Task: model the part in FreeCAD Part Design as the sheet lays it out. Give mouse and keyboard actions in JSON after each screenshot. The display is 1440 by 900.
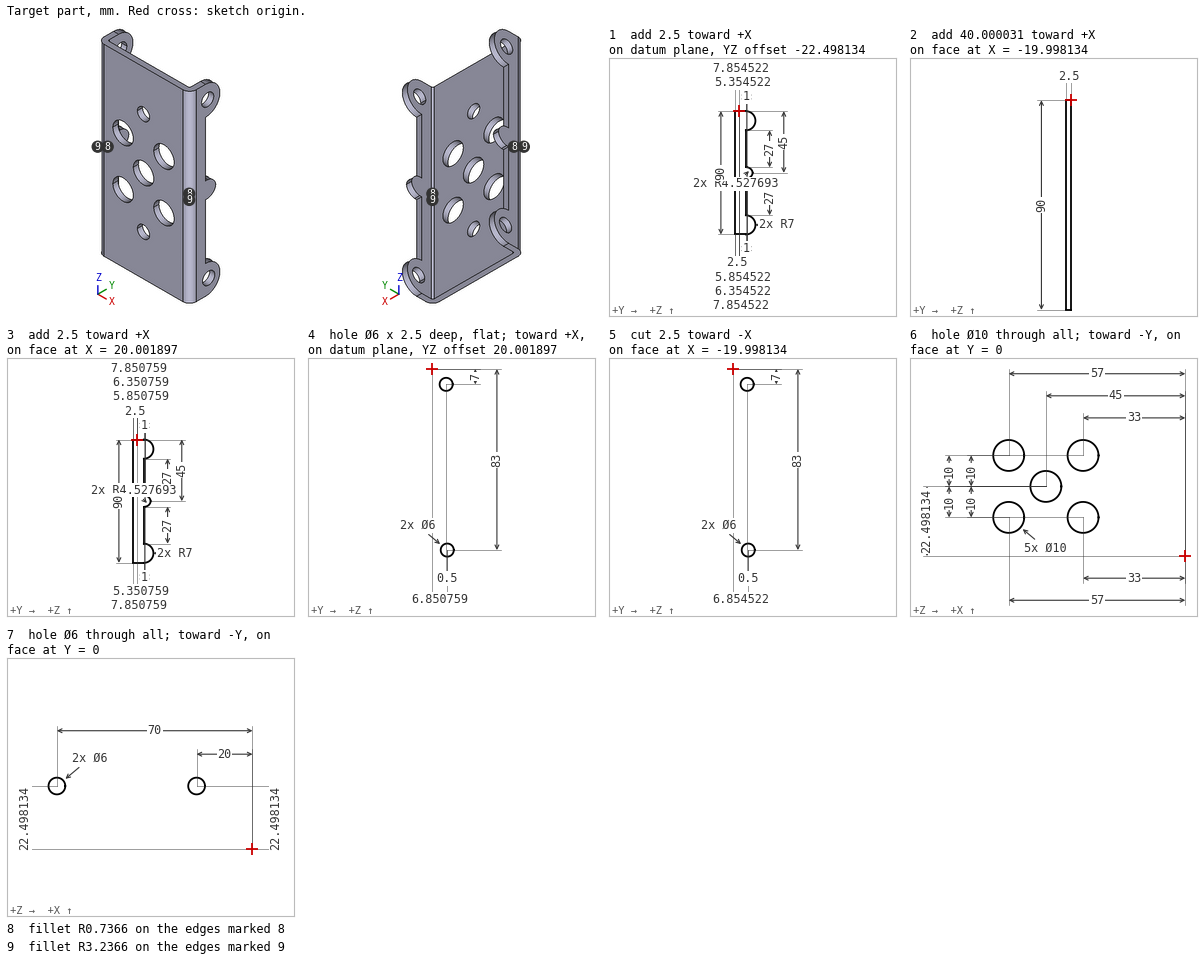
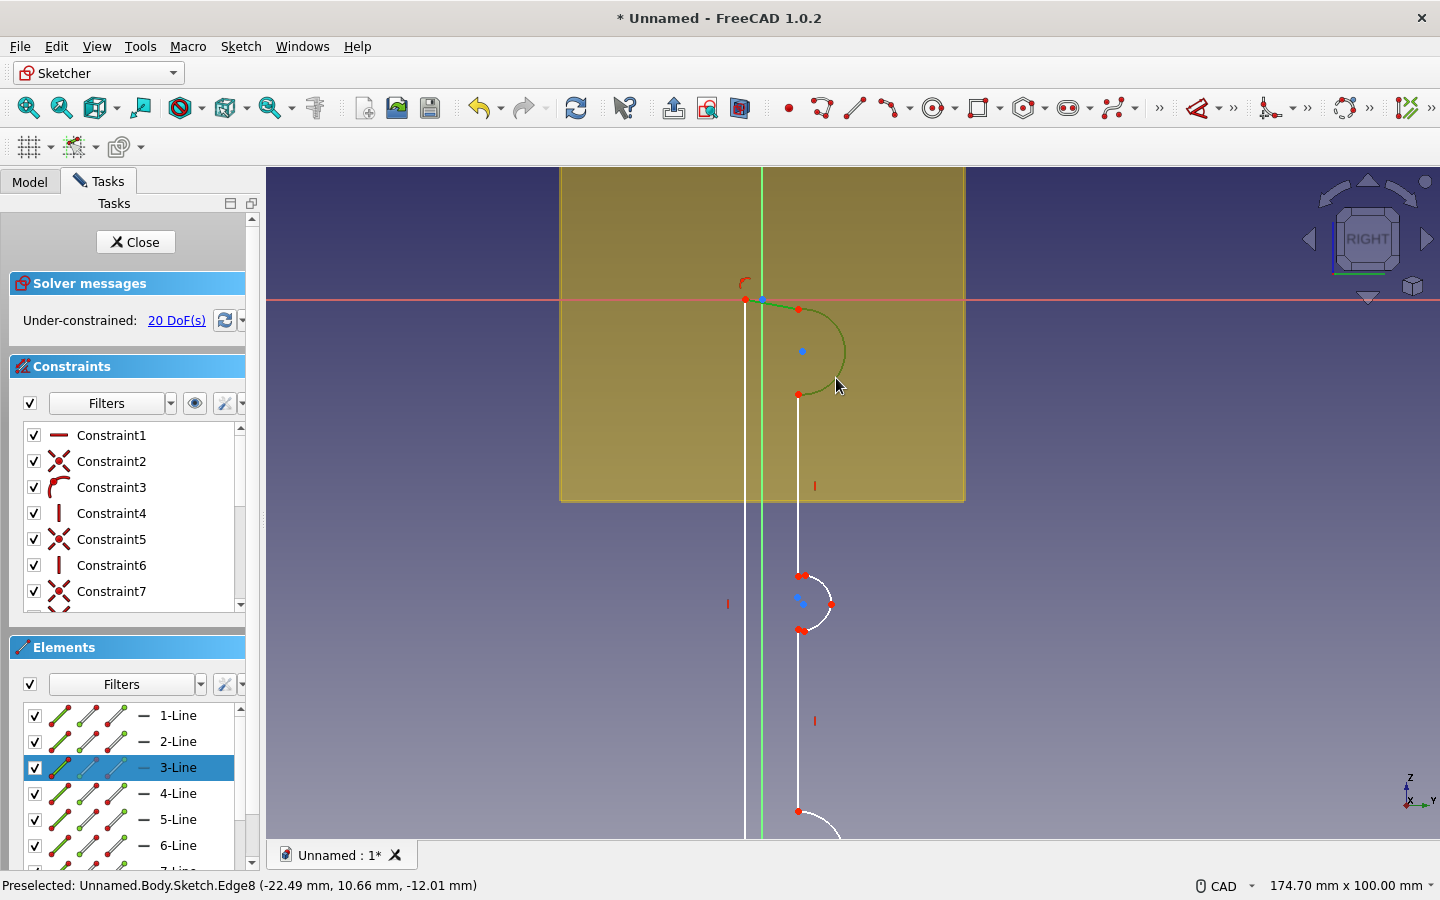
{"action": "key", "text": "t"}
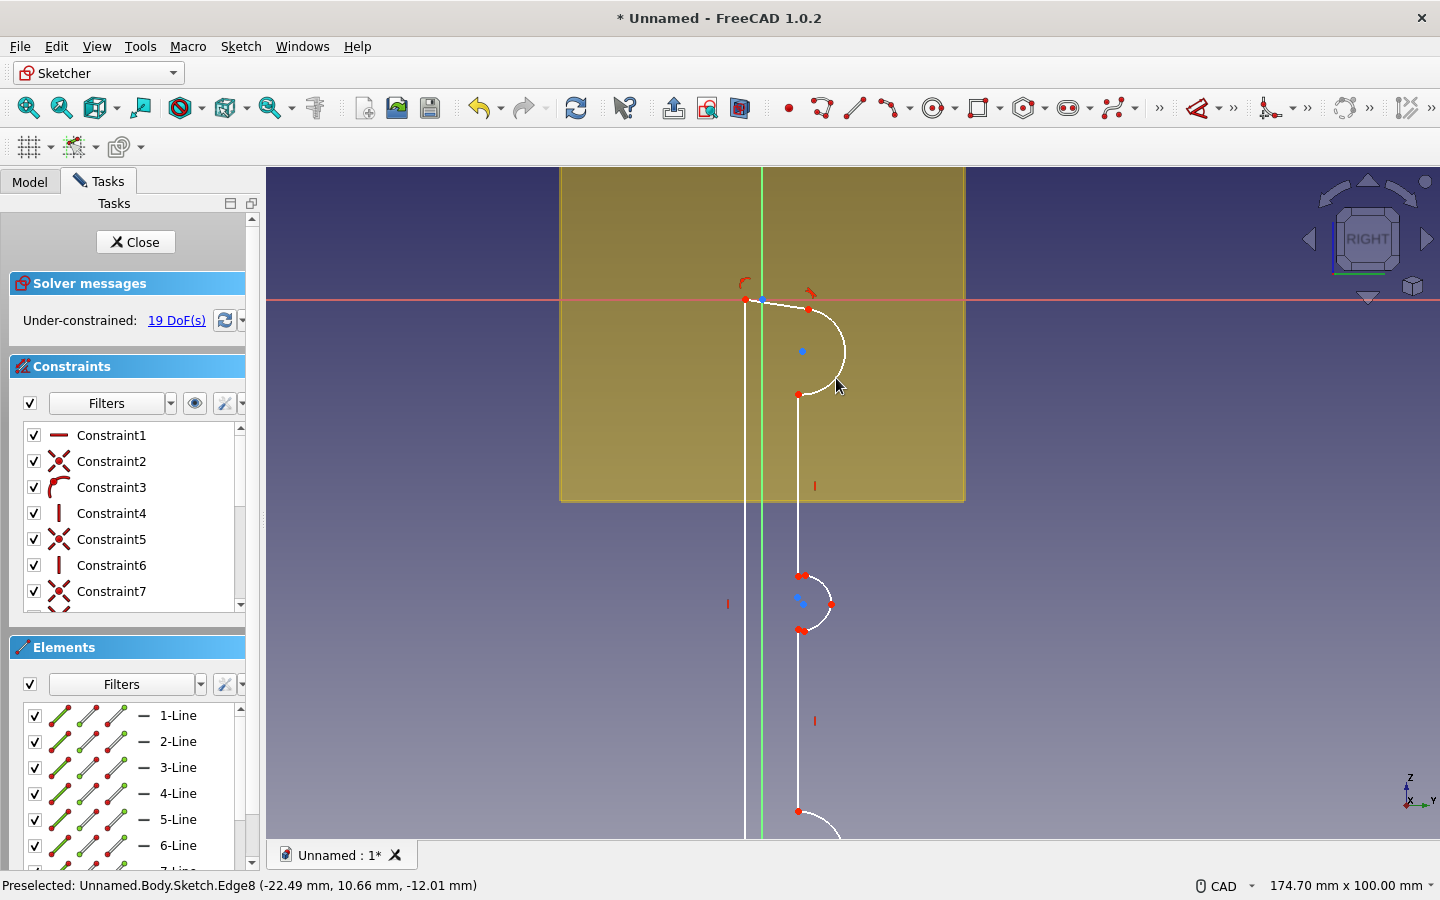
{"action": "left_click", "coordinate": [771, 304]}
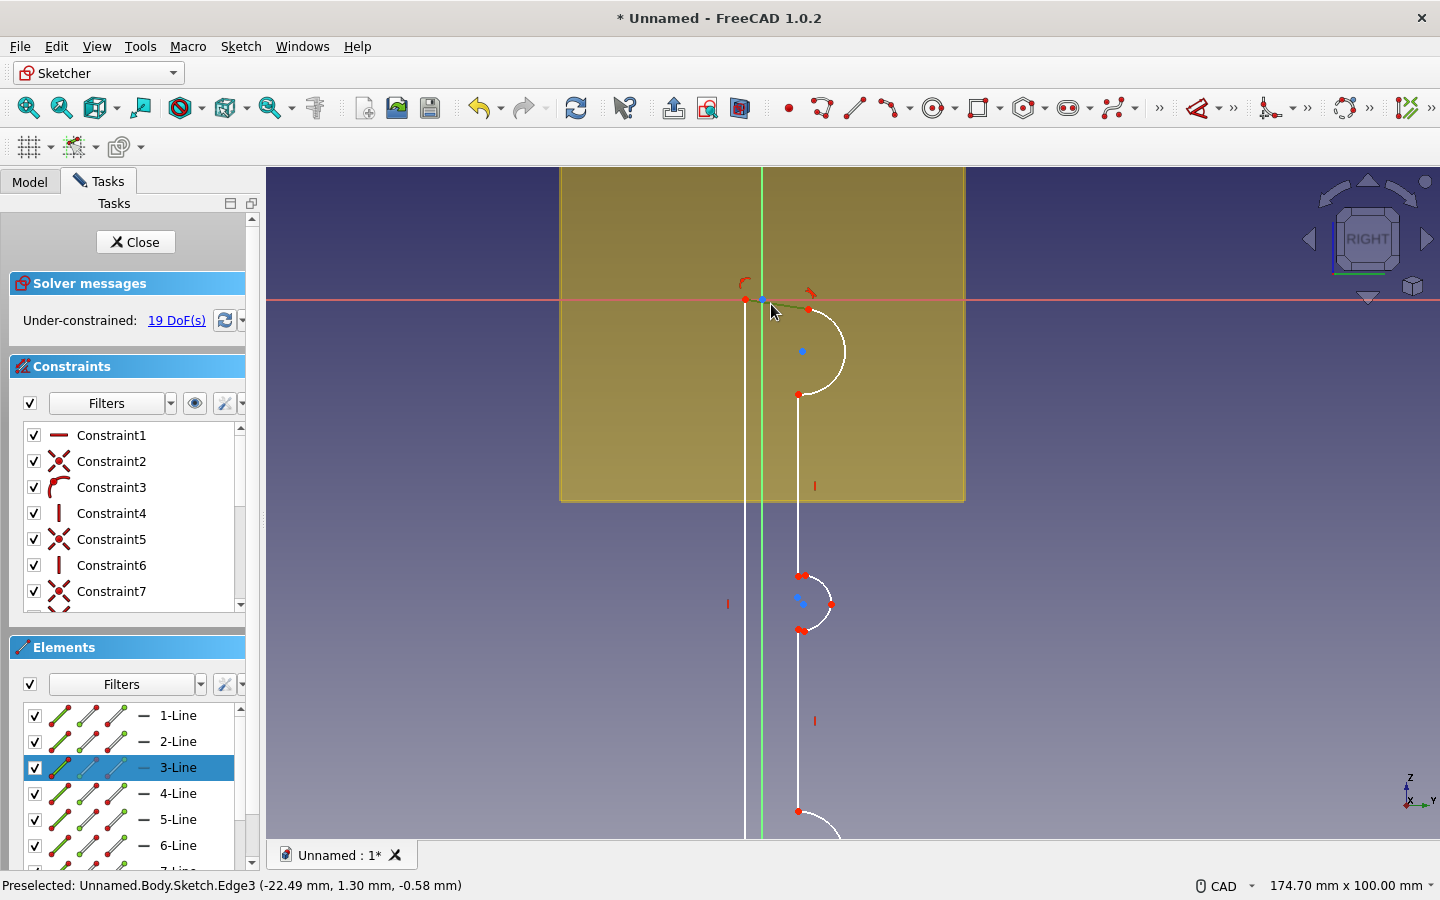
{"action": "key", "text": "h"}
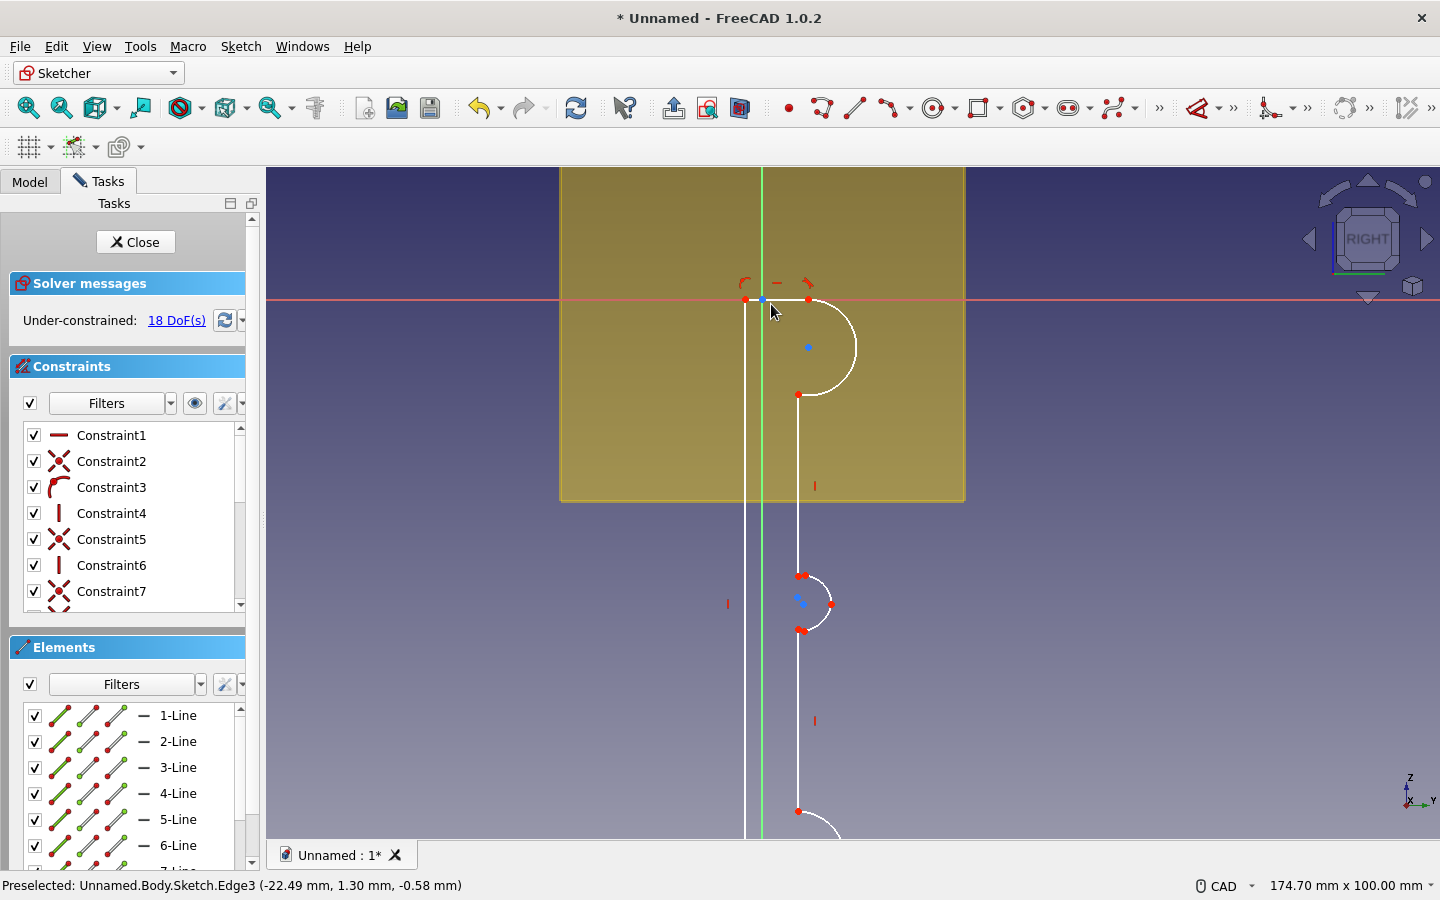
{"action": "scroll", "coordinate": [802, 576], "scroll_direction": "up", "scroll_amount": 7}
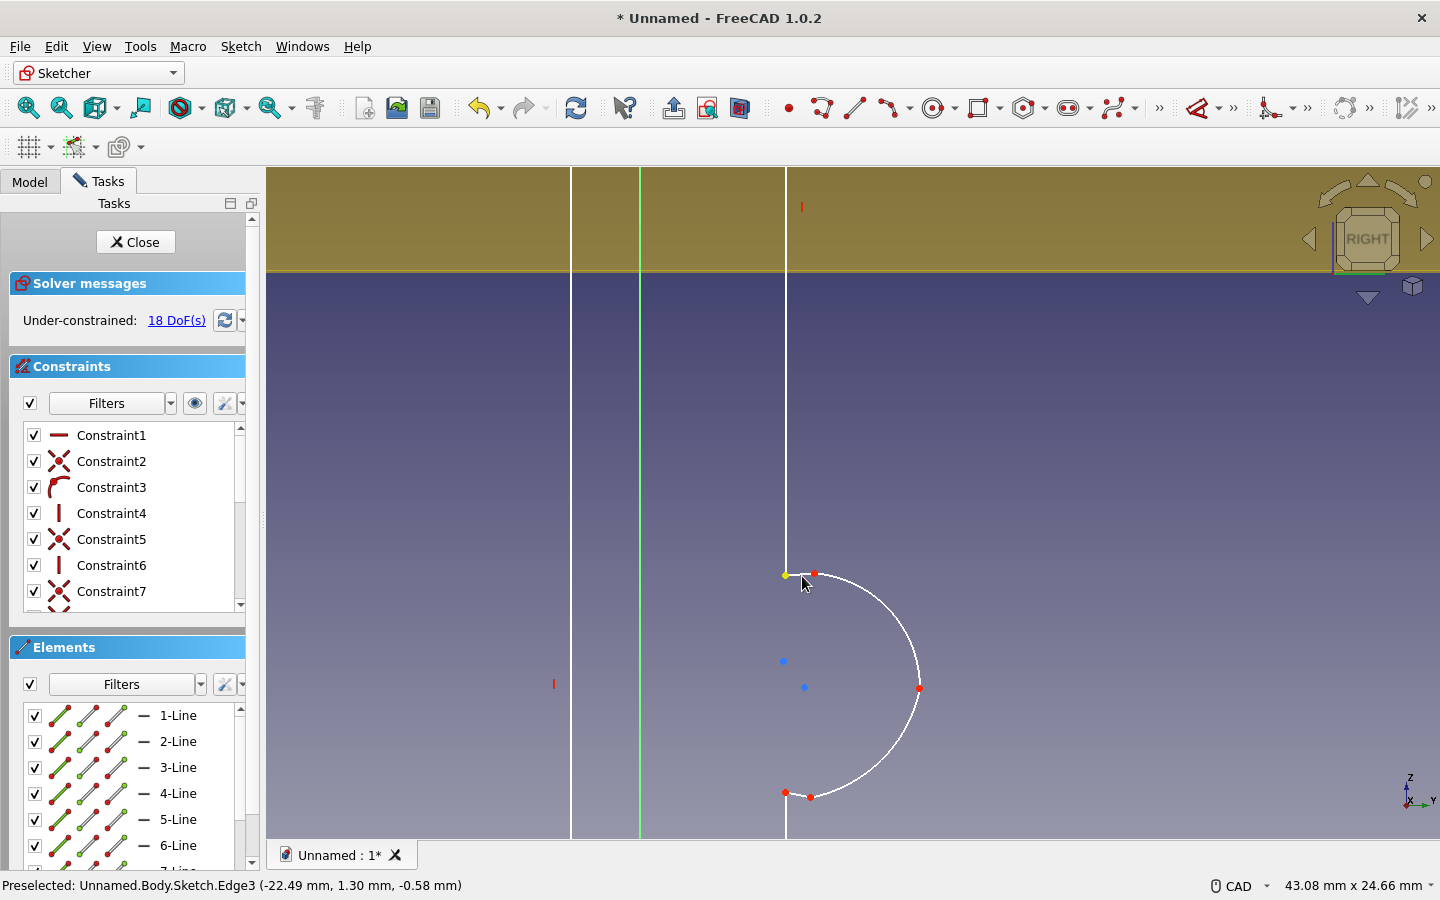
{"action": "left_click", "coordinate": [800, 574]}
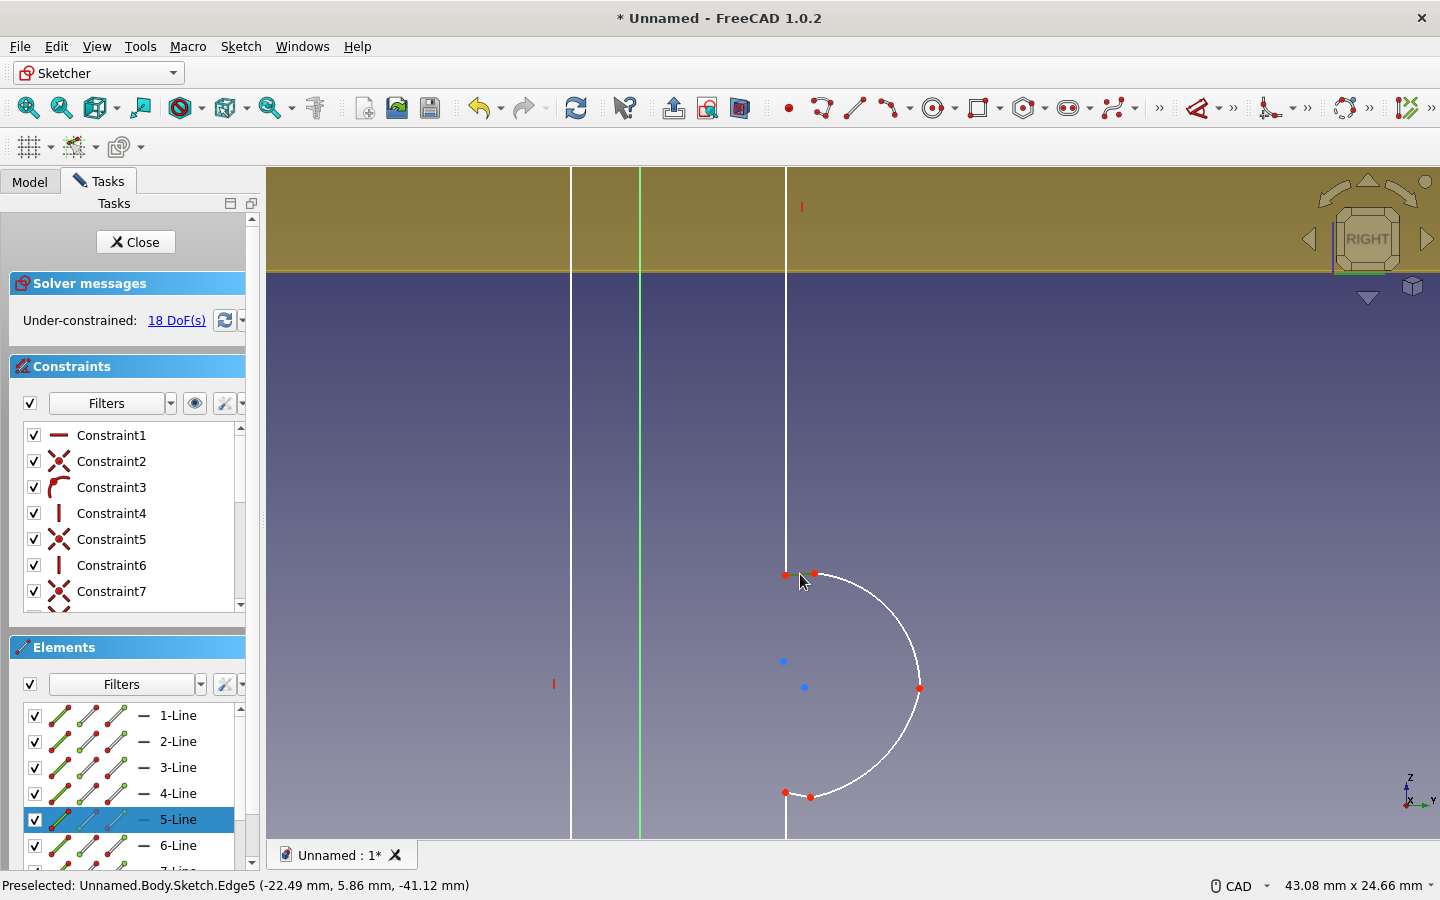
{"action": "key", "text": "h"}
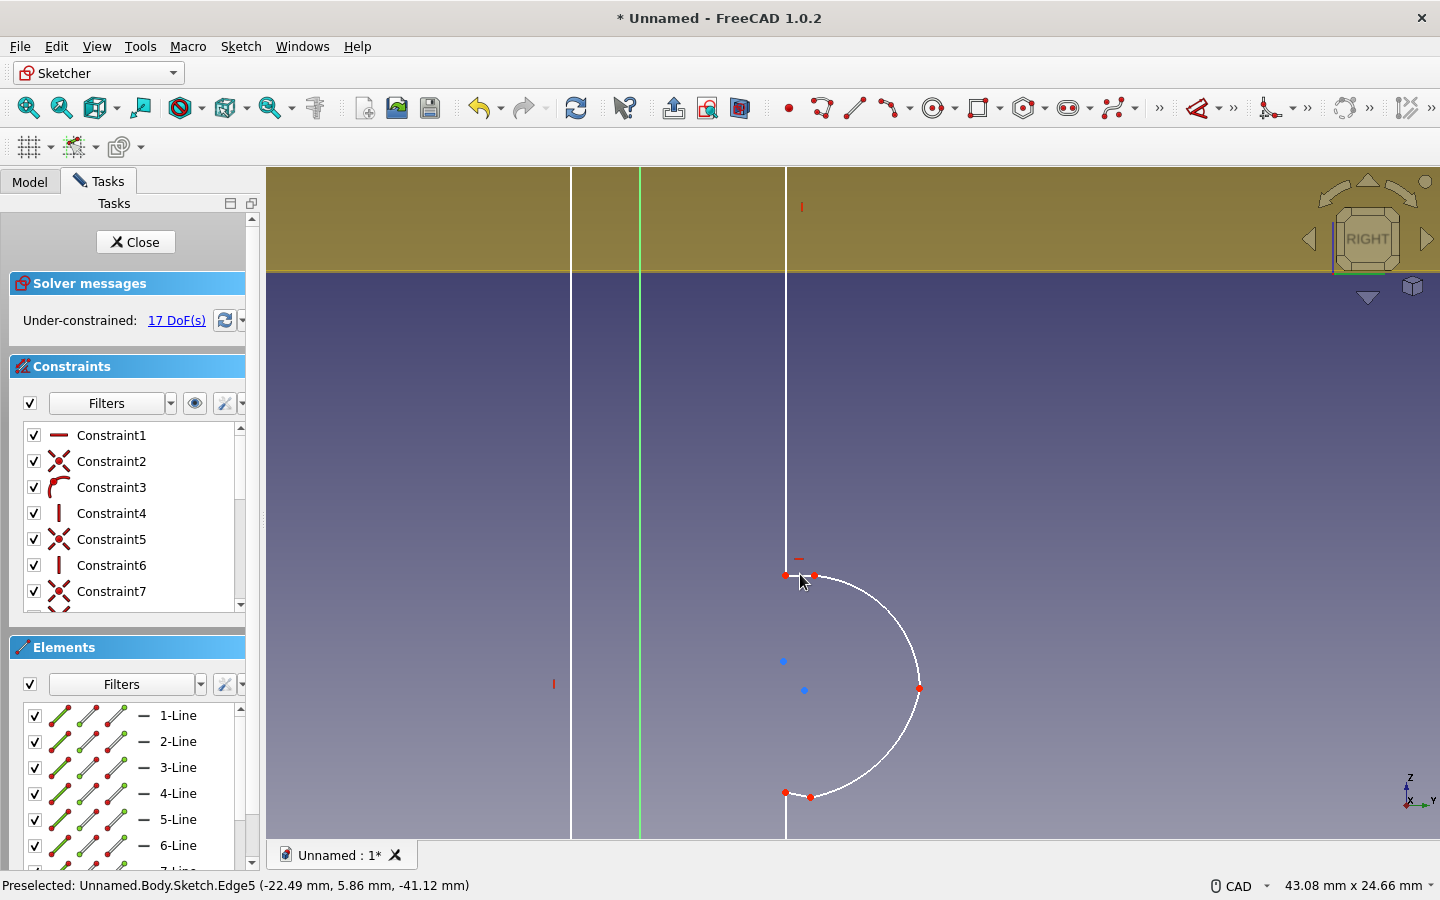
{"action": "scroll", "coordinate": [801, 796], "scroll_direction": "up", "scroll_amount": 2}